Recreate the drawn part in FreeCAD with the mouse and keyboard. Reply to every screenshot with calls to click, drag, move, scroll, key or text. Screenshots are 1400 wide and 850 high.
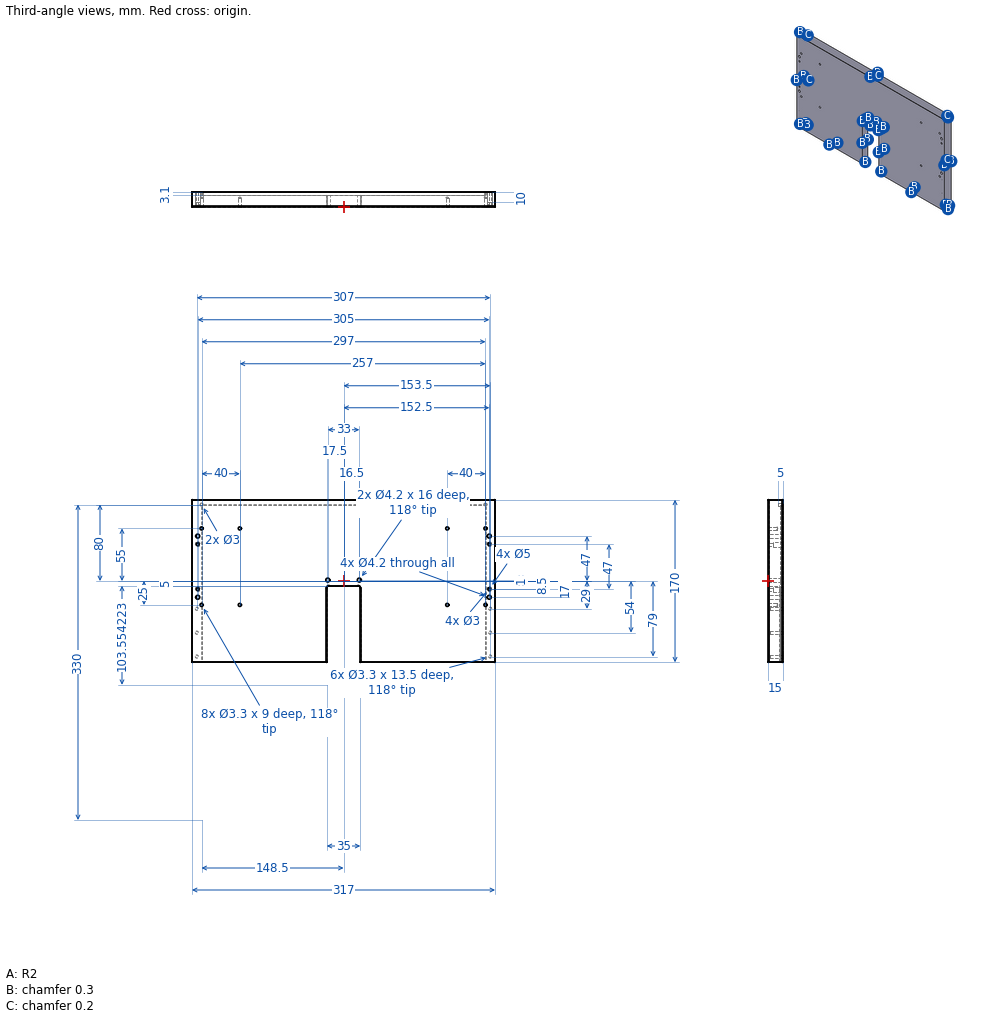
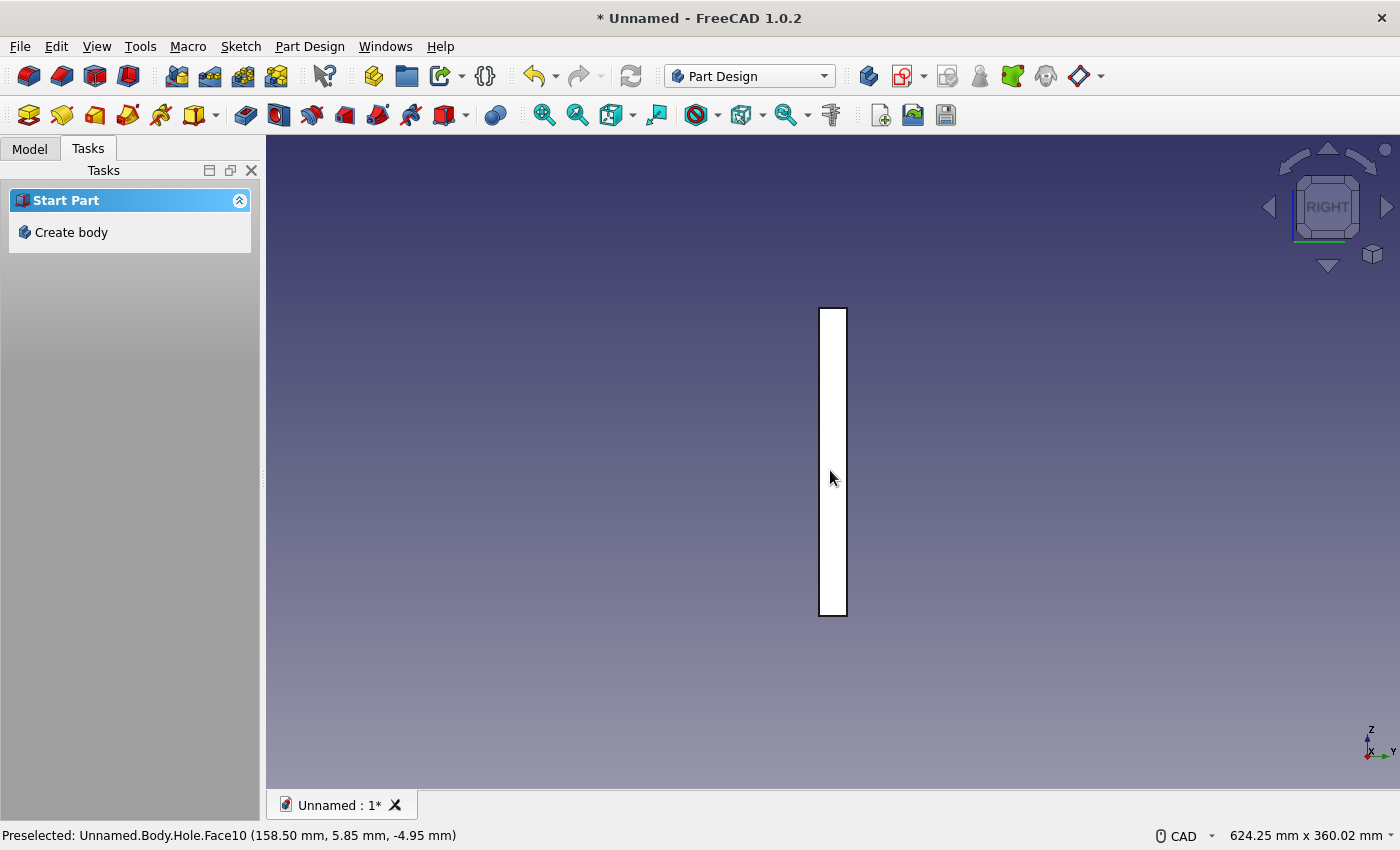
key(5)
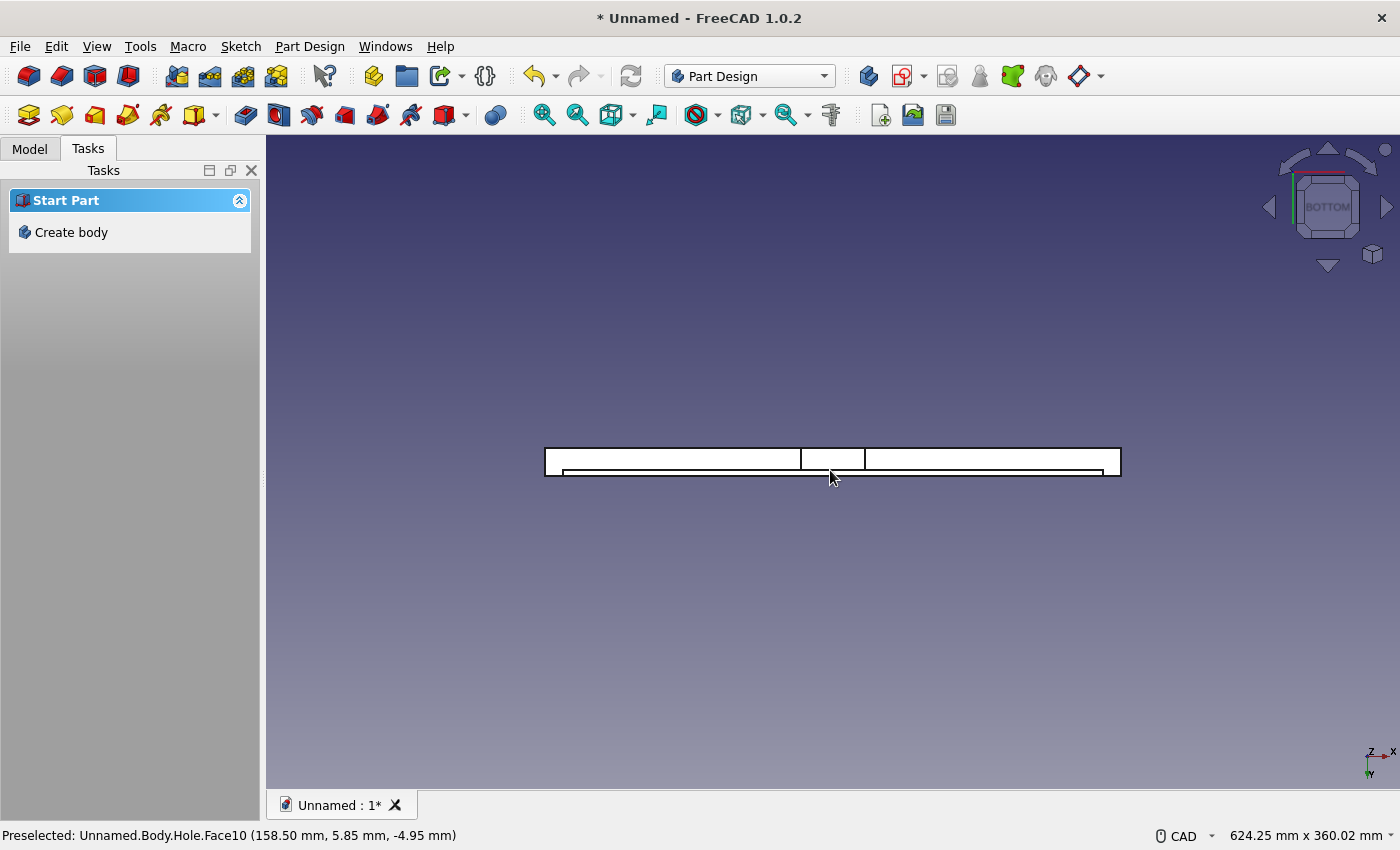
scroll(865, 458, up, 4)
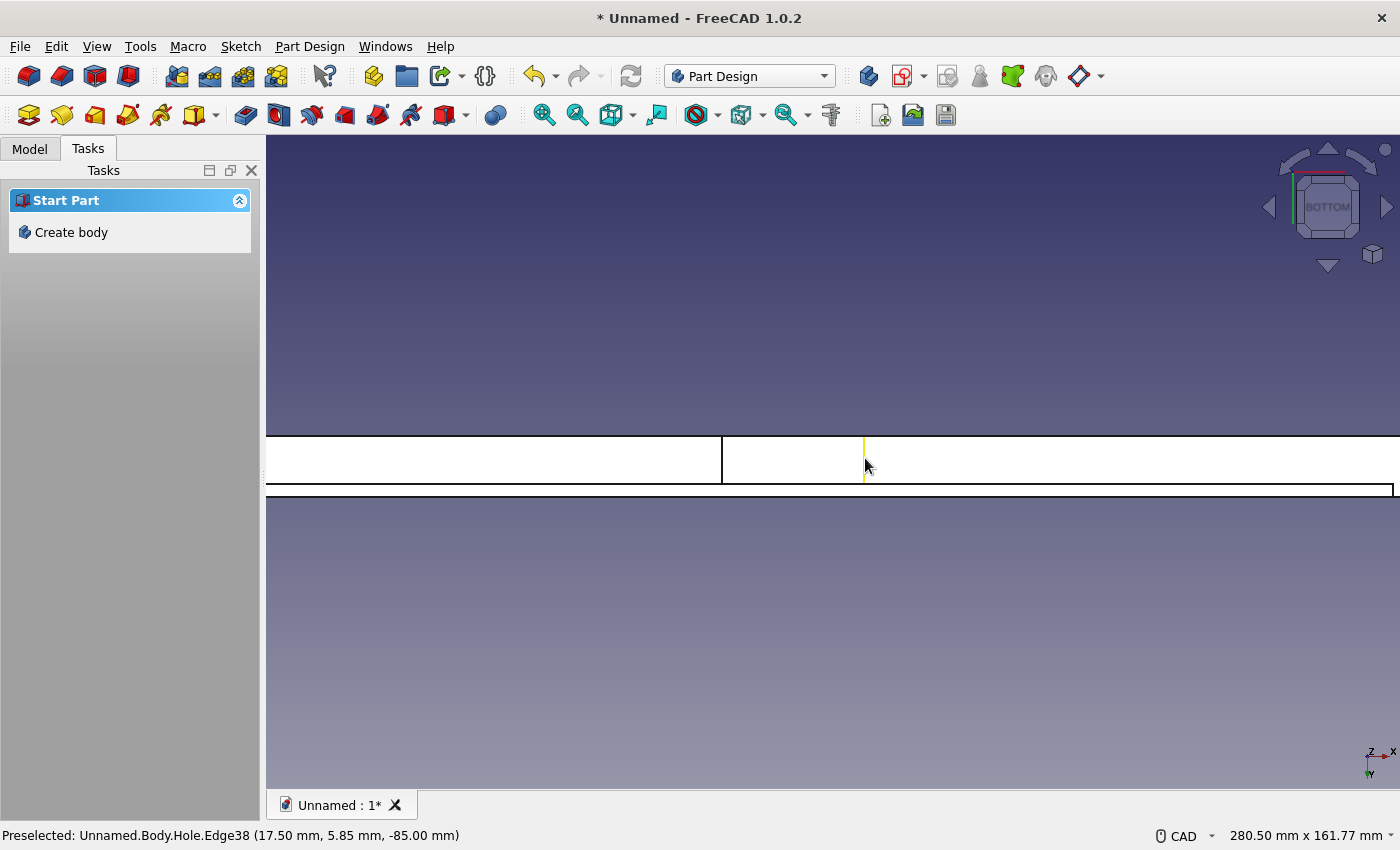
click(545, 116)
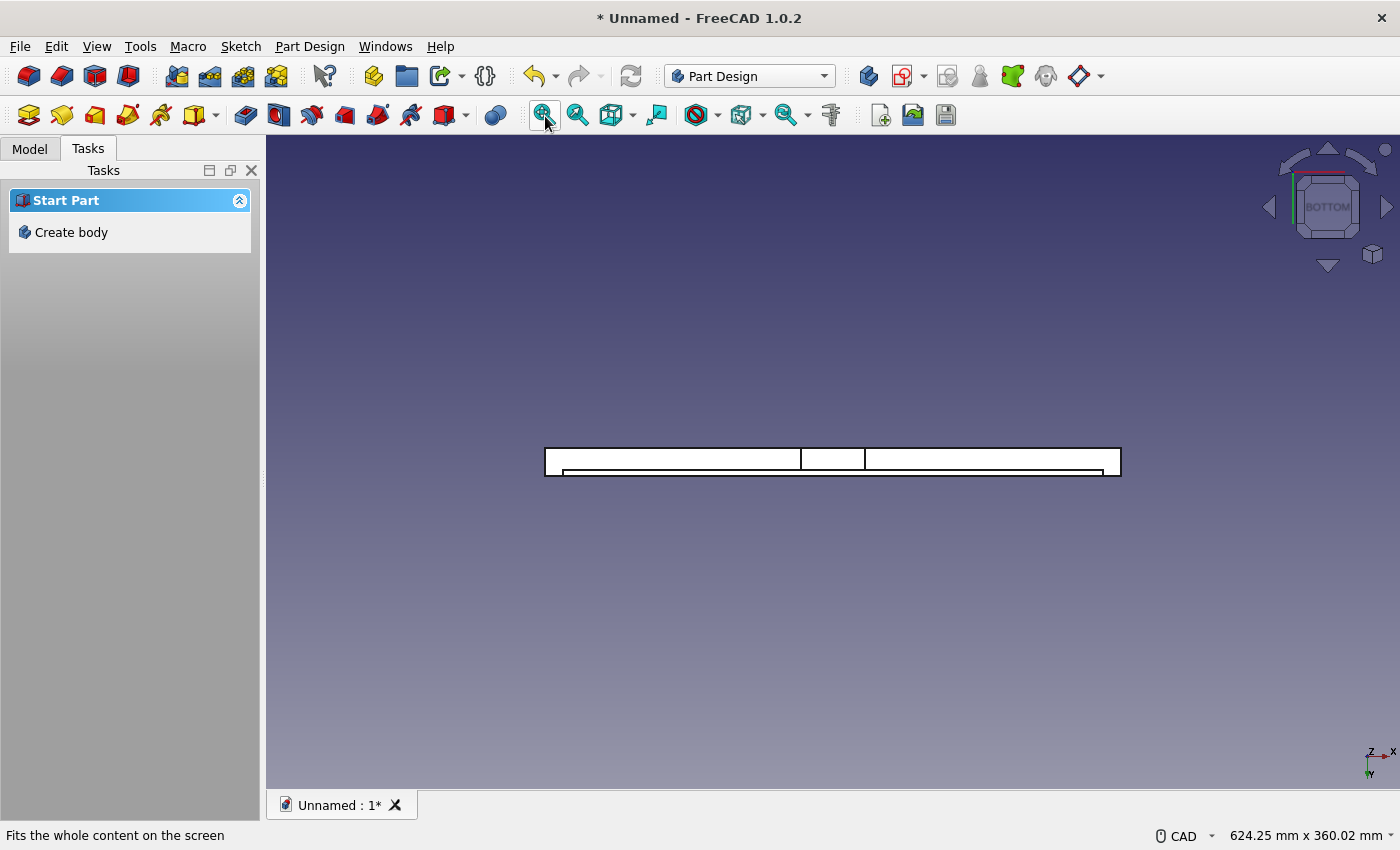
key(4)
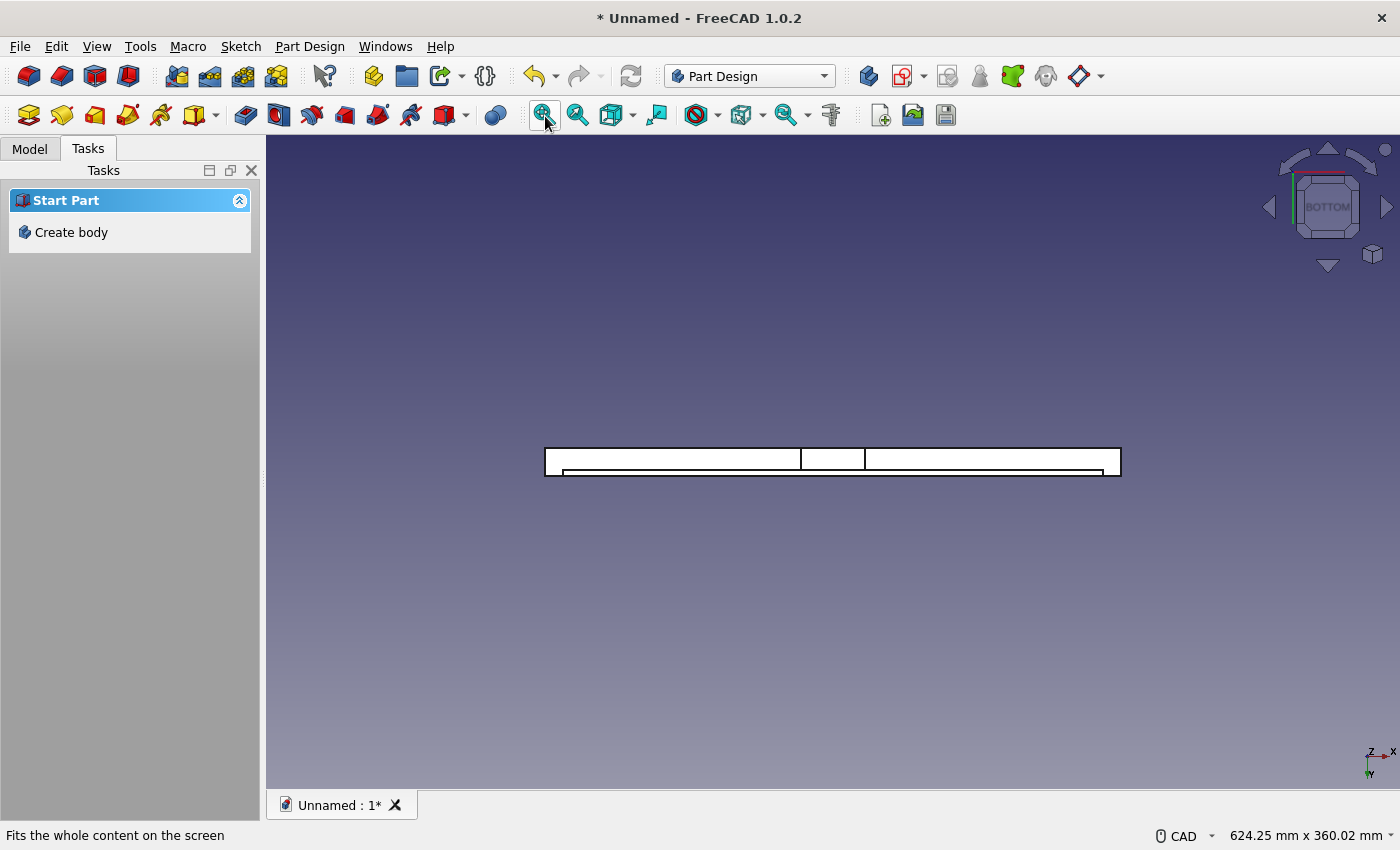
scroll(801, 470, up, 4)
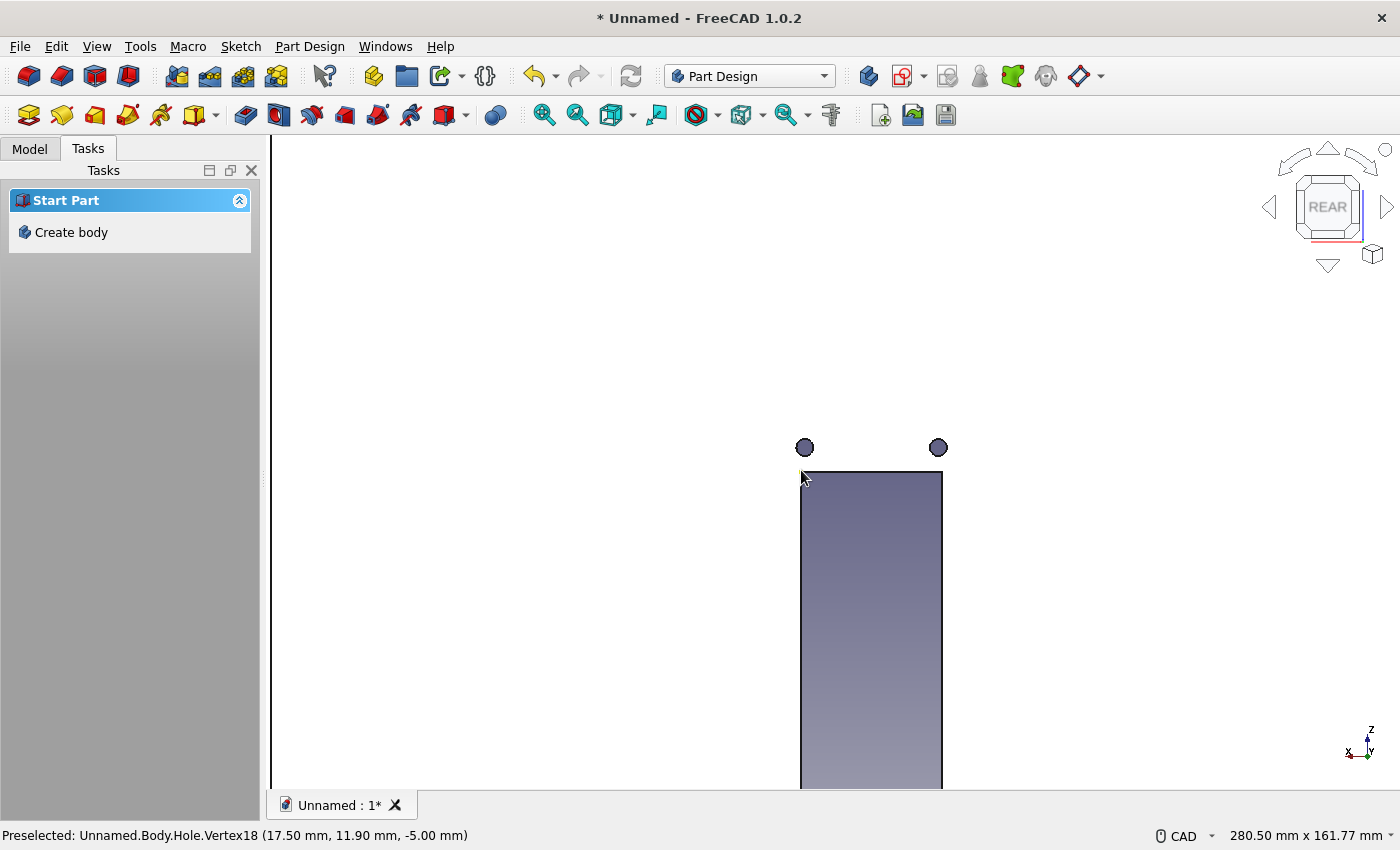
key(v)
key(f)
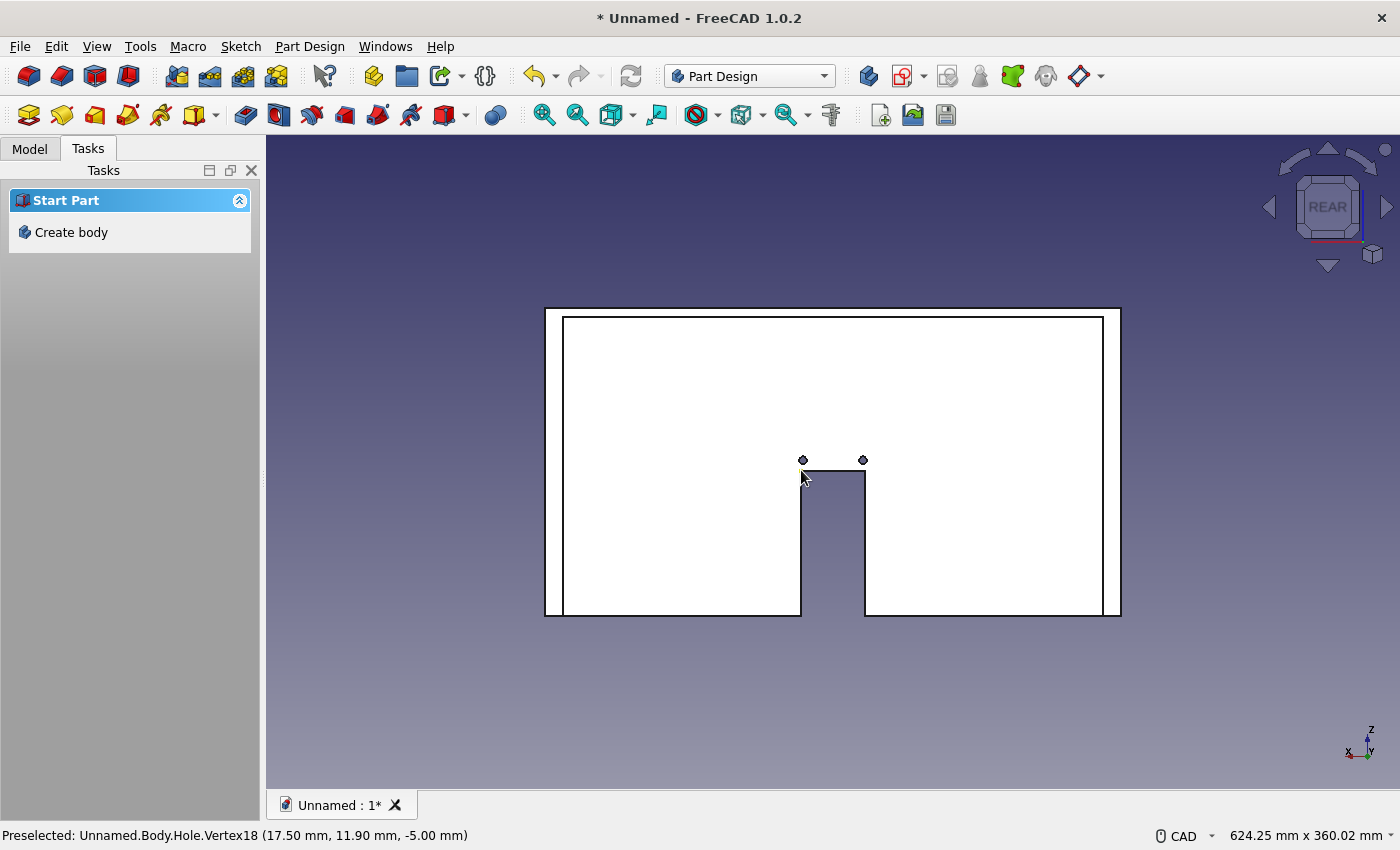
key(6)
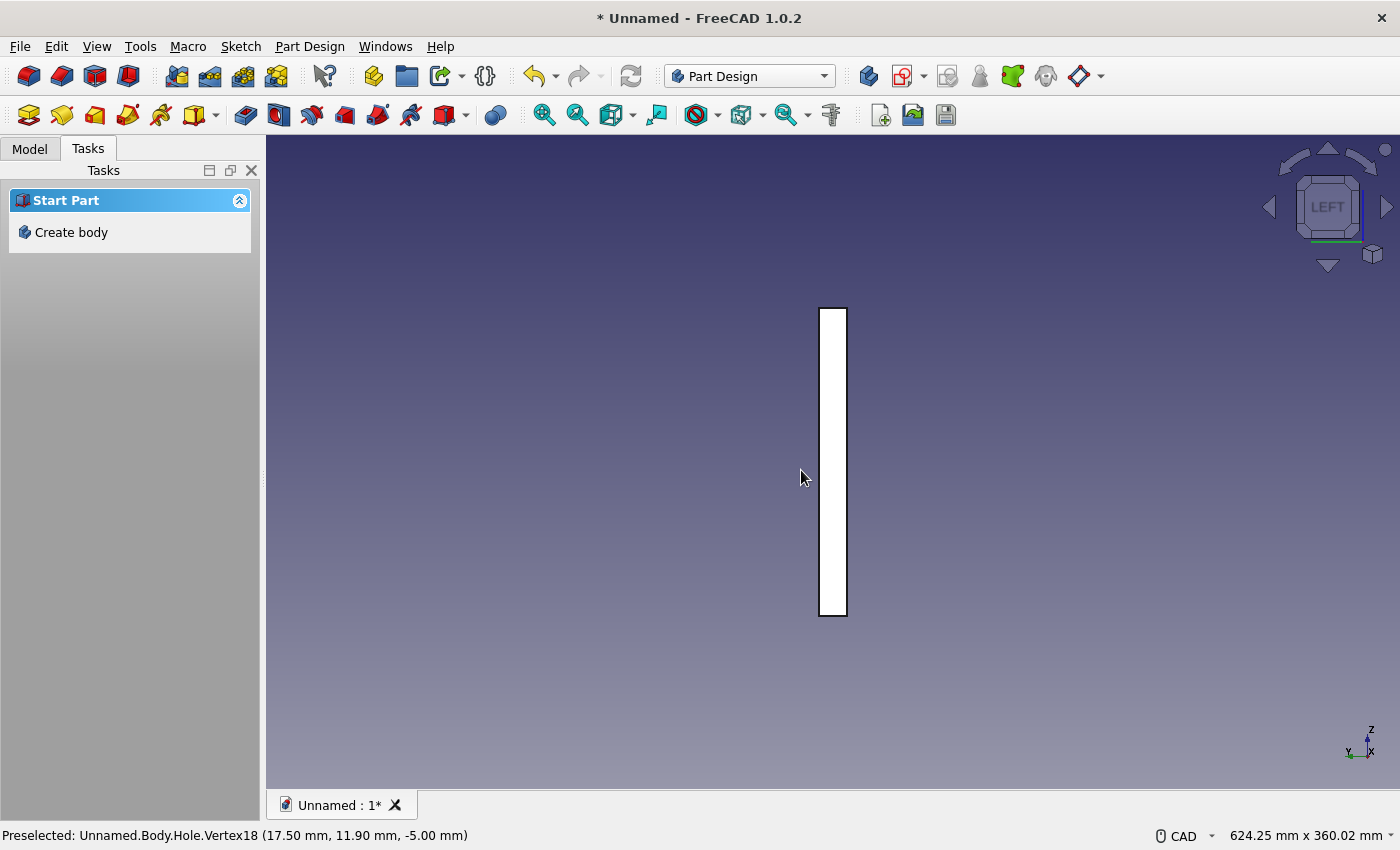
scroll(836, 470, up, 4)